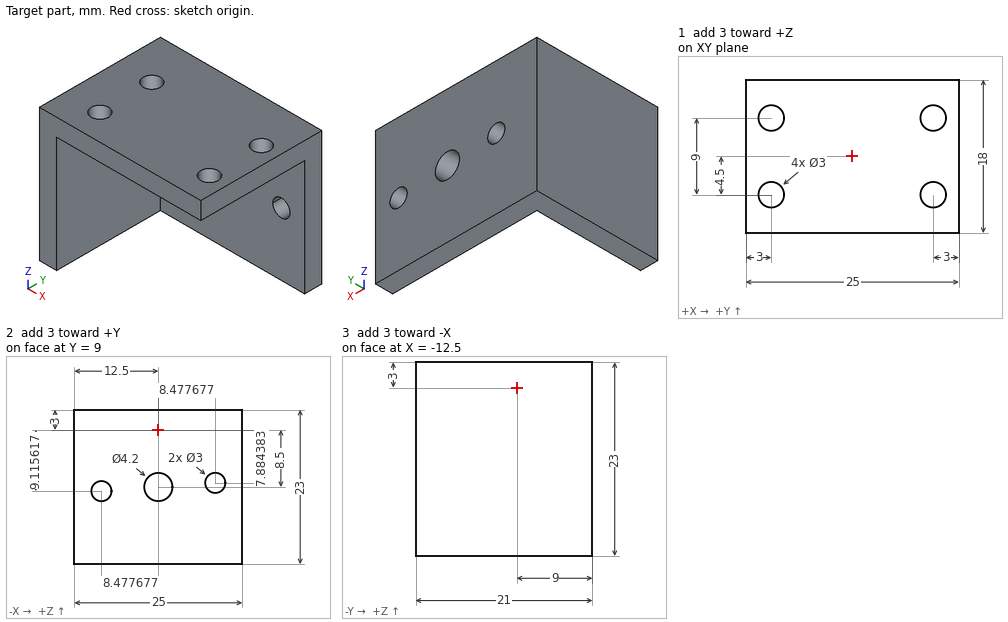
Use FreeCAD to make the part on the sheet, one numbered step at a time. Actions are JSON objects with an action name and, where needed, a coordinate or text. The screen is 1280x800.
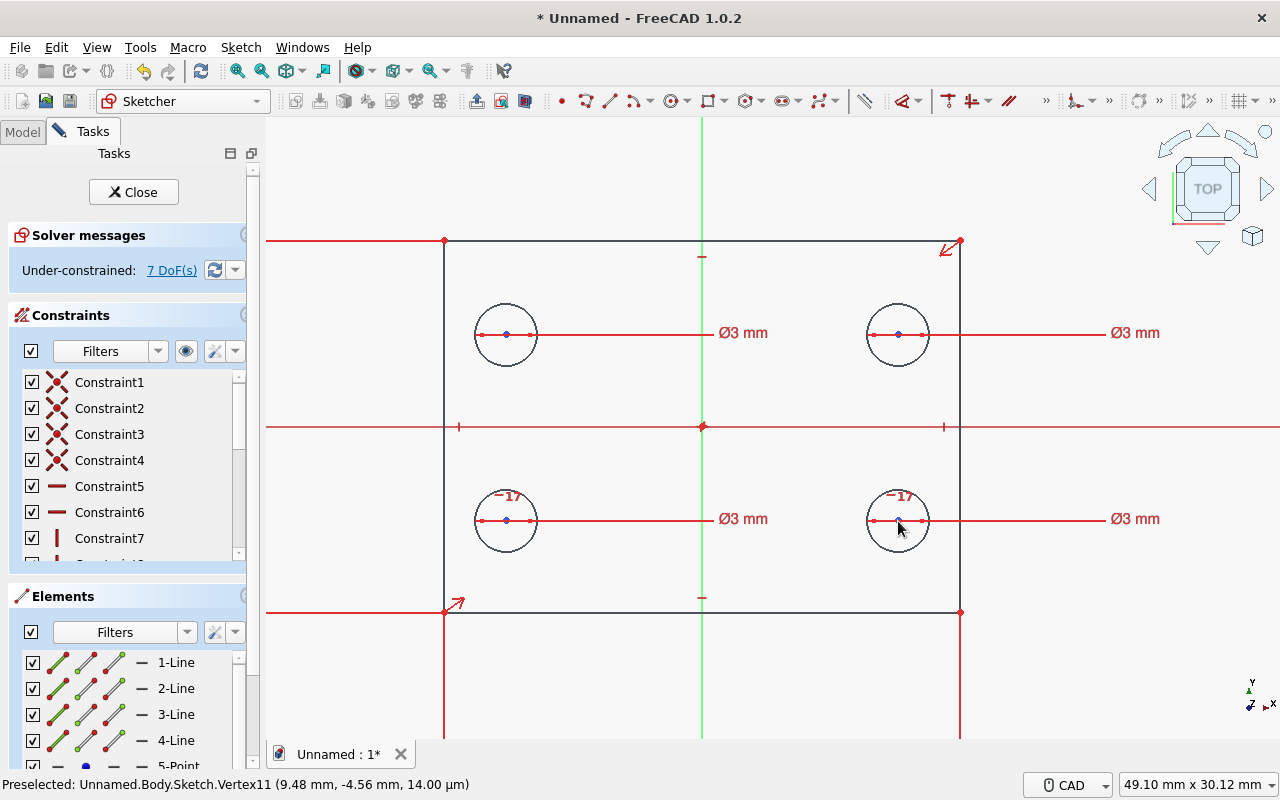
{"action": "left_click", "coordinate": [506, 521]}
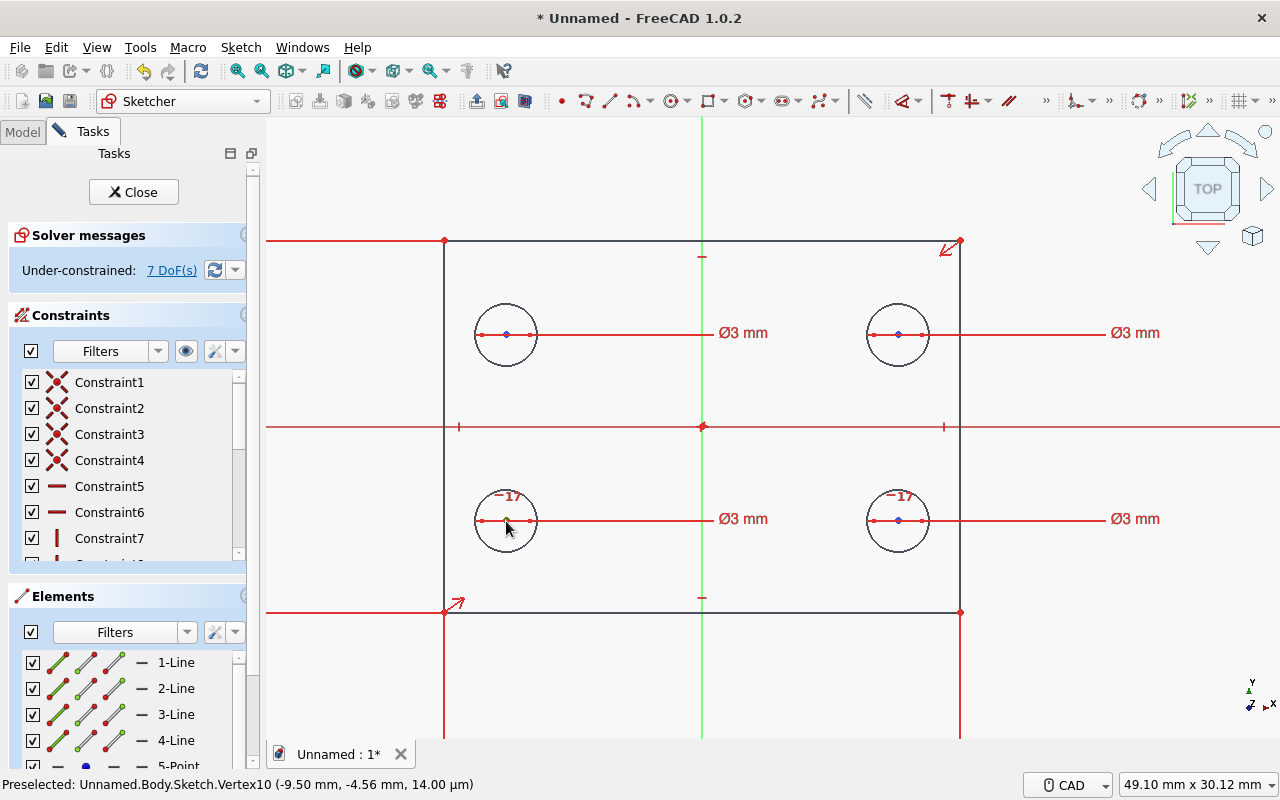
{"action": "left_click", "coordinate": [506, 335]}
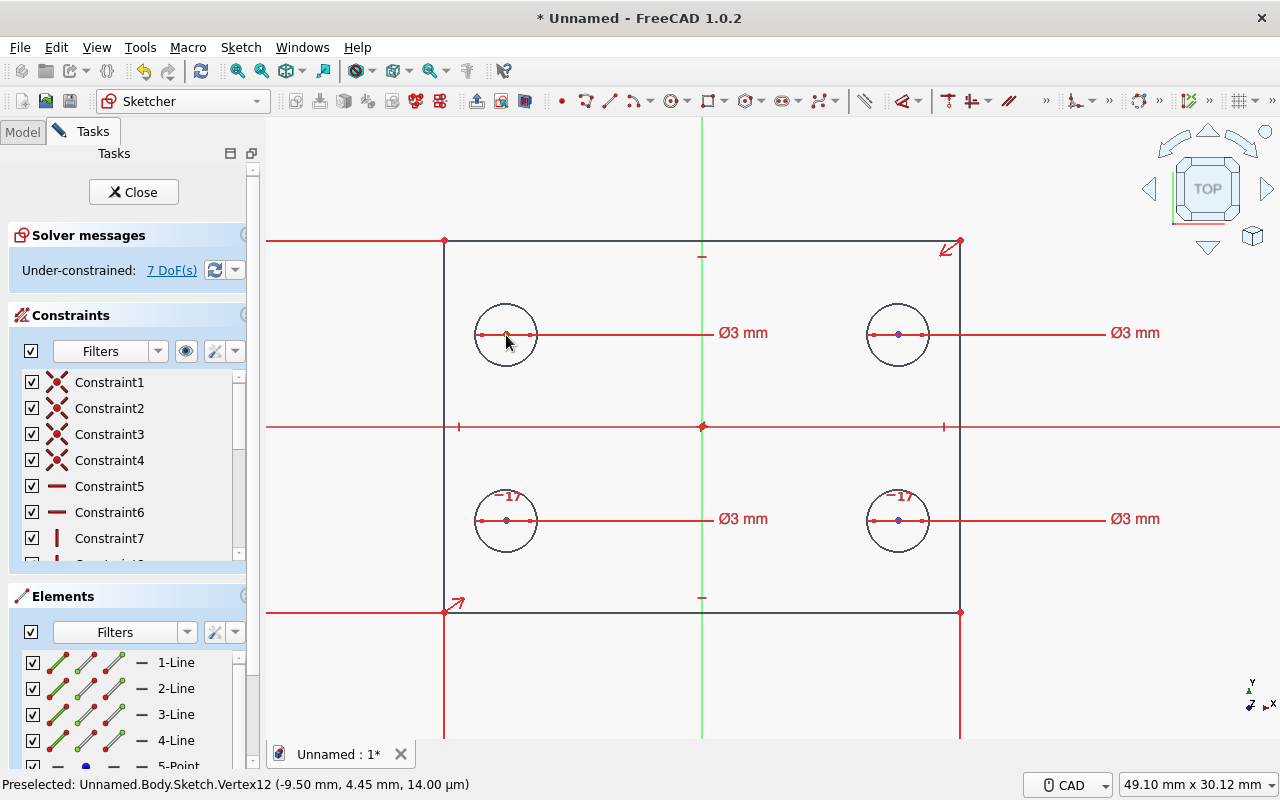
{"action": "left_click", "coordinate": [990, 102]}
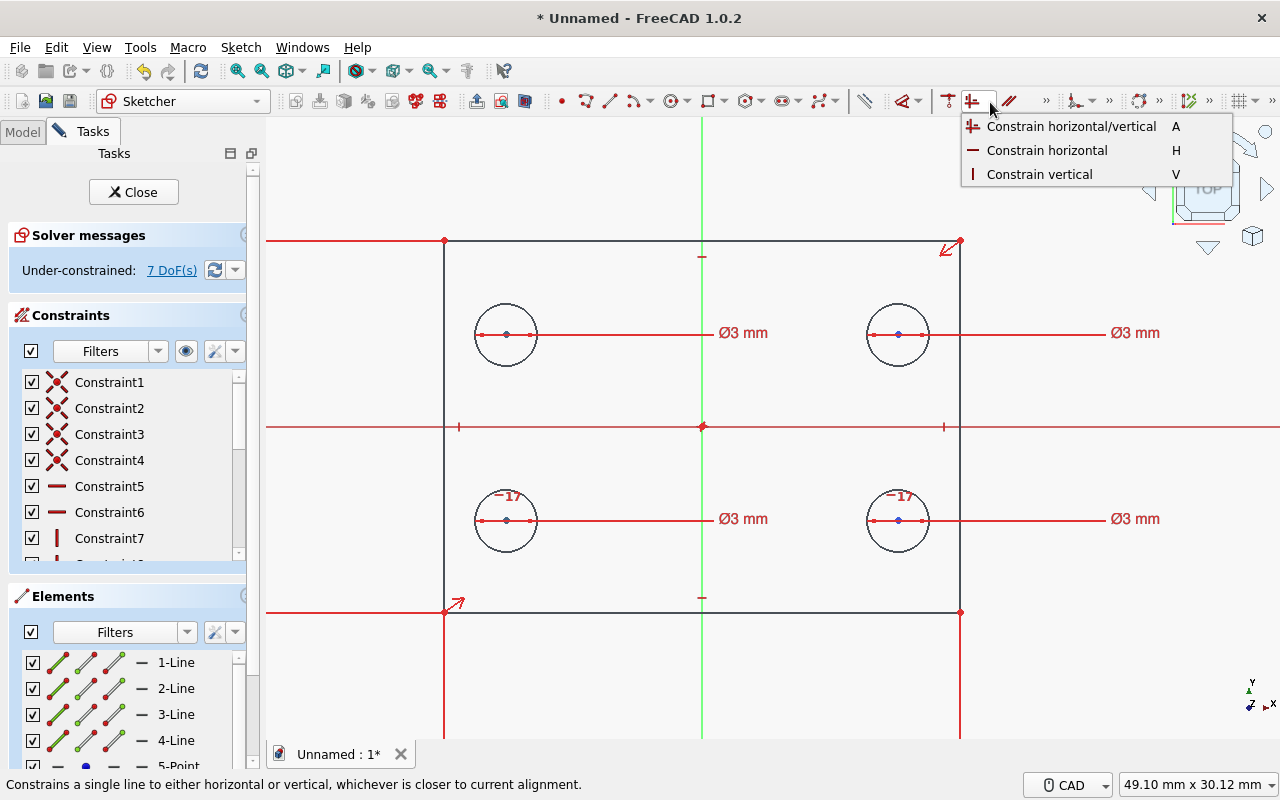
{"action": "left_click", "coordinate": [1097, 174]}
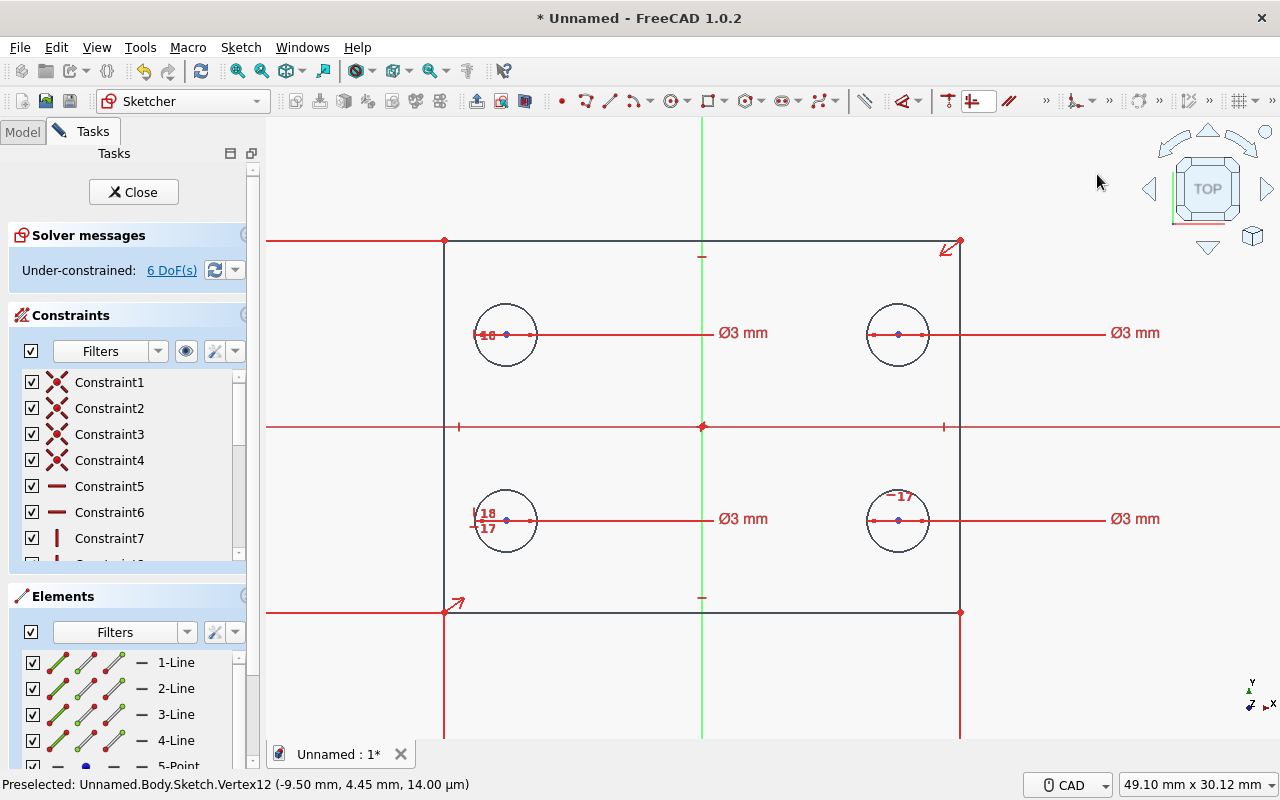
{"action": "left_click", "coordinate": [898, 521]}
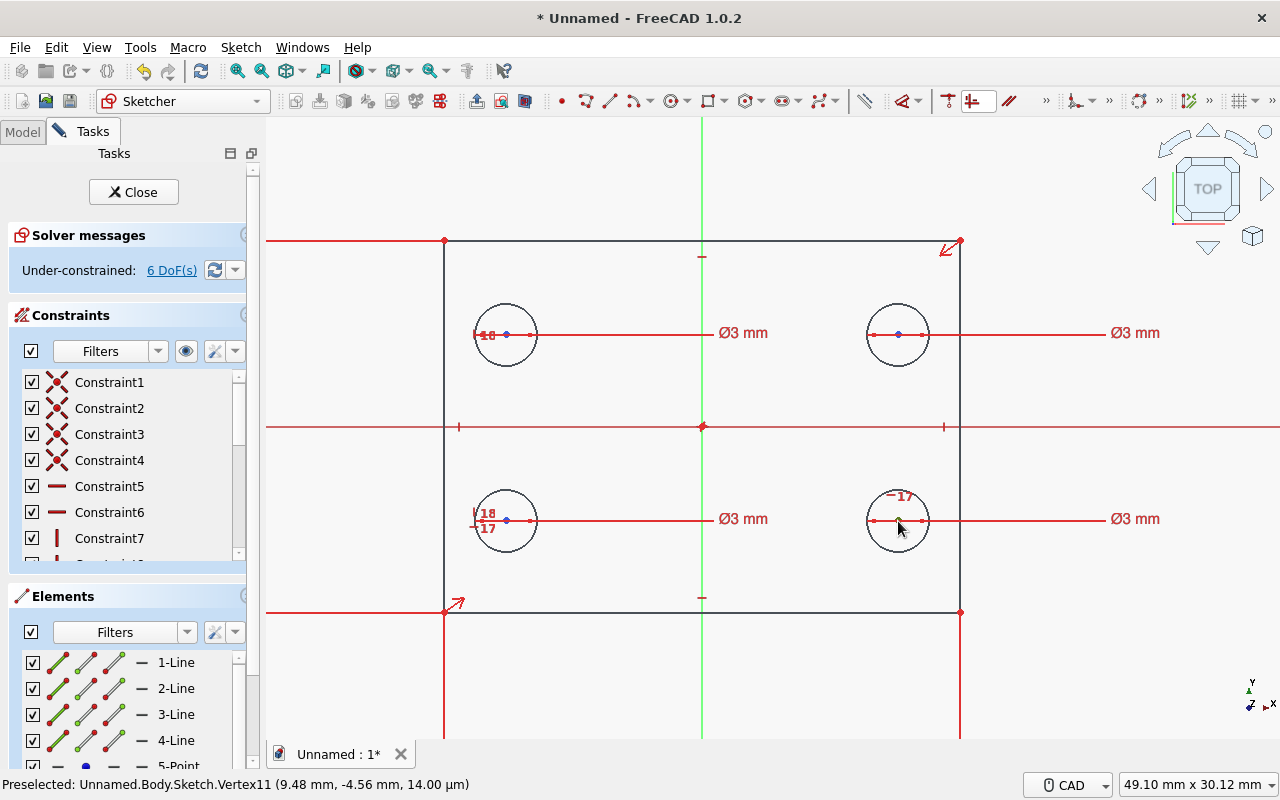
{"action": "left_click", "coordinate": [898, 335]}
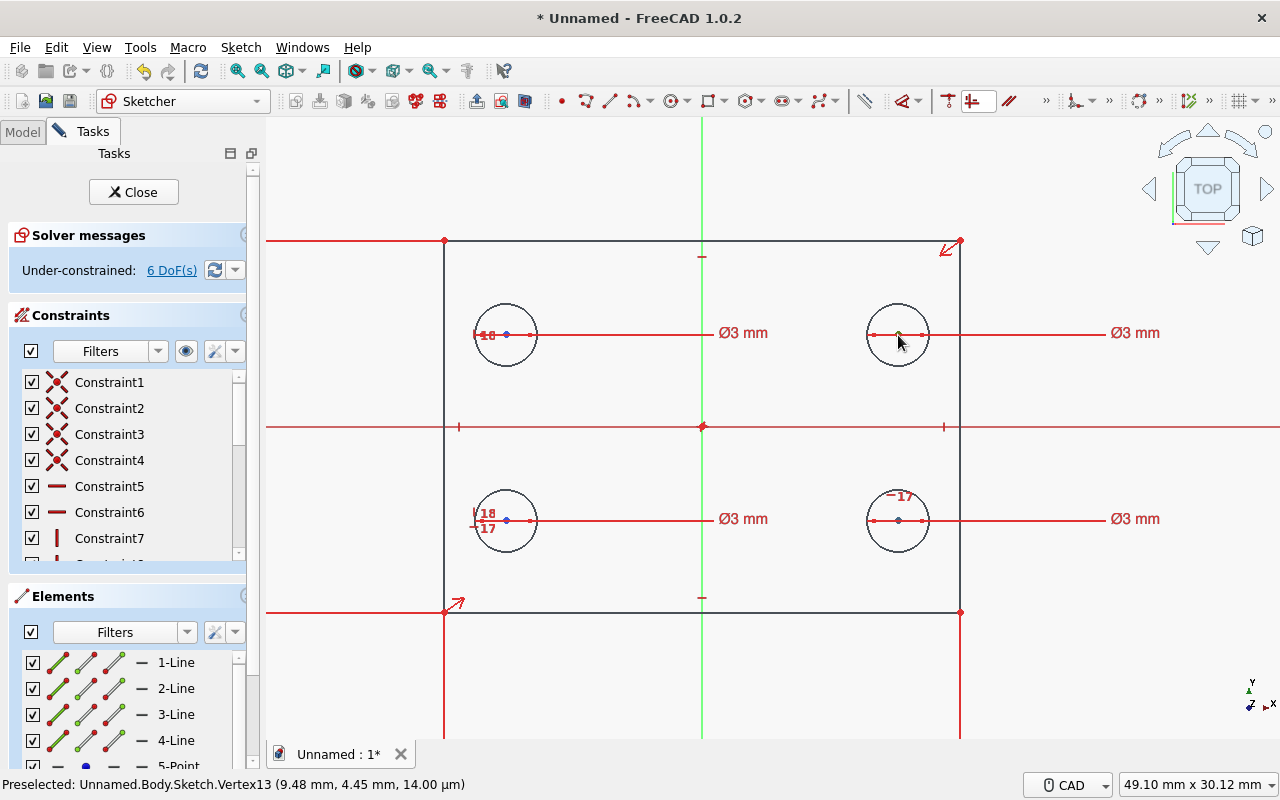
{"action": "key", "text": "v"}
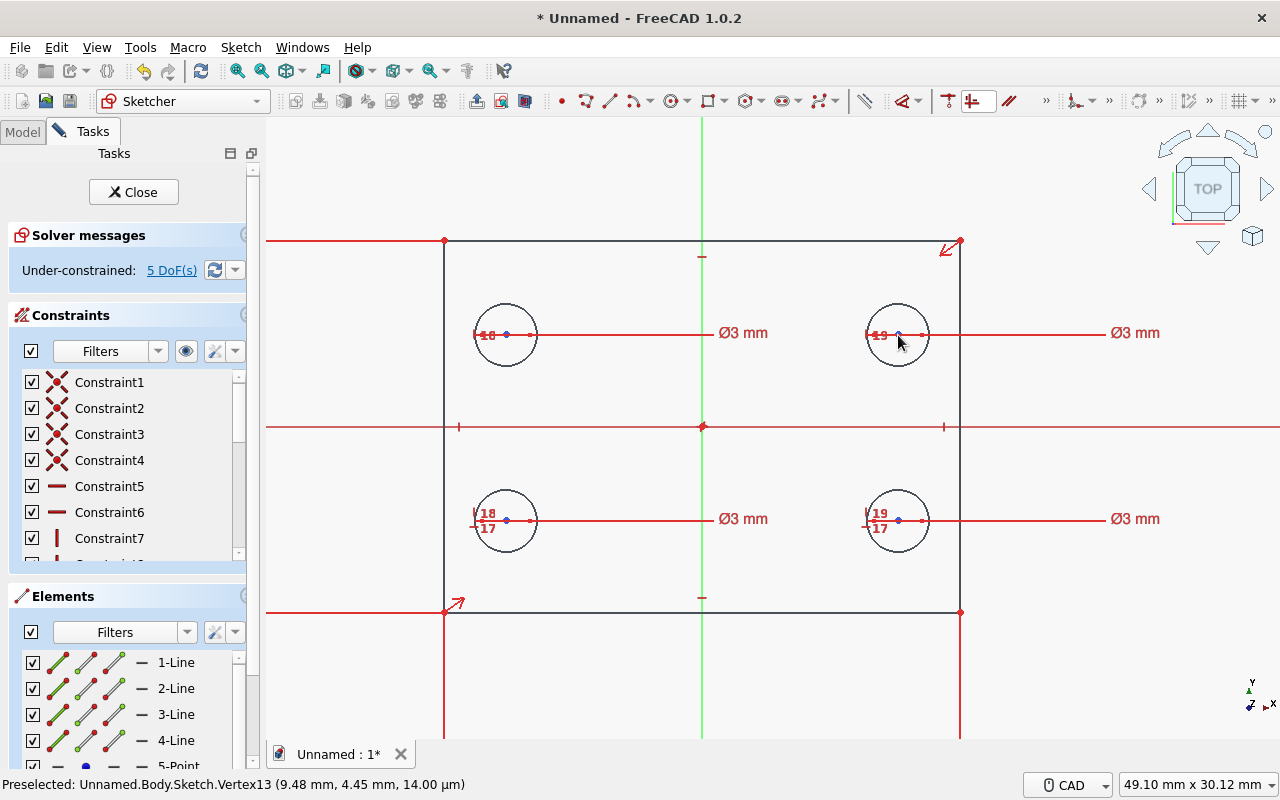
{"action": "left_click", "coordinate": [506, 335]}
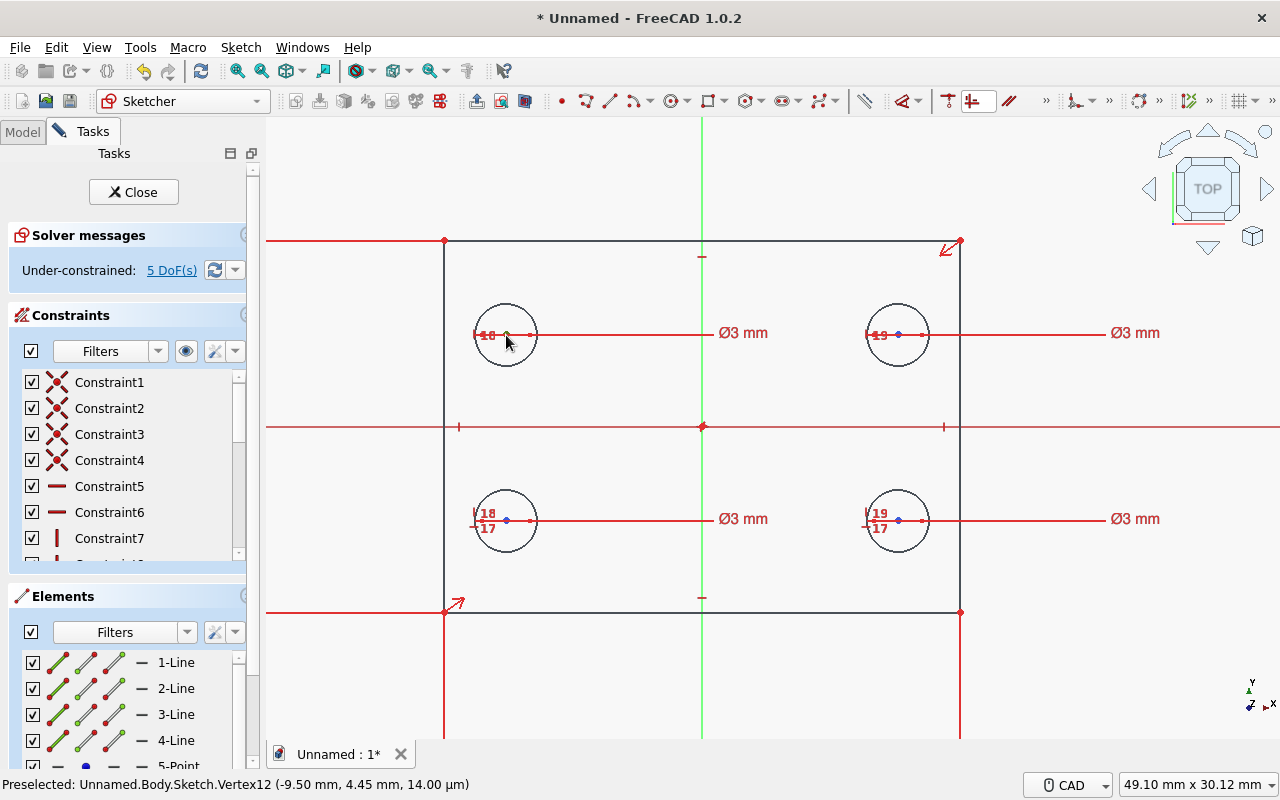
{"action": "left_click", "coordinate": [898, 335]}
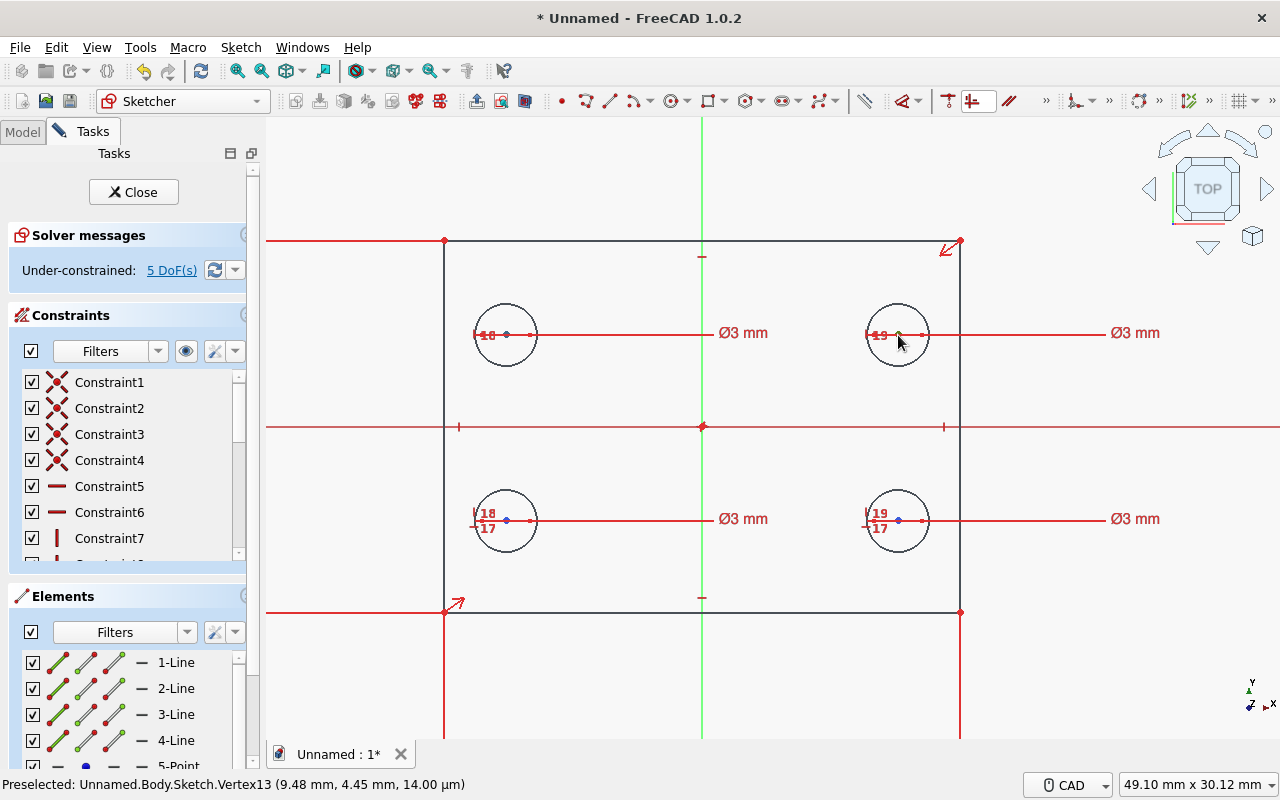
{"action": "key", "text": "h"}